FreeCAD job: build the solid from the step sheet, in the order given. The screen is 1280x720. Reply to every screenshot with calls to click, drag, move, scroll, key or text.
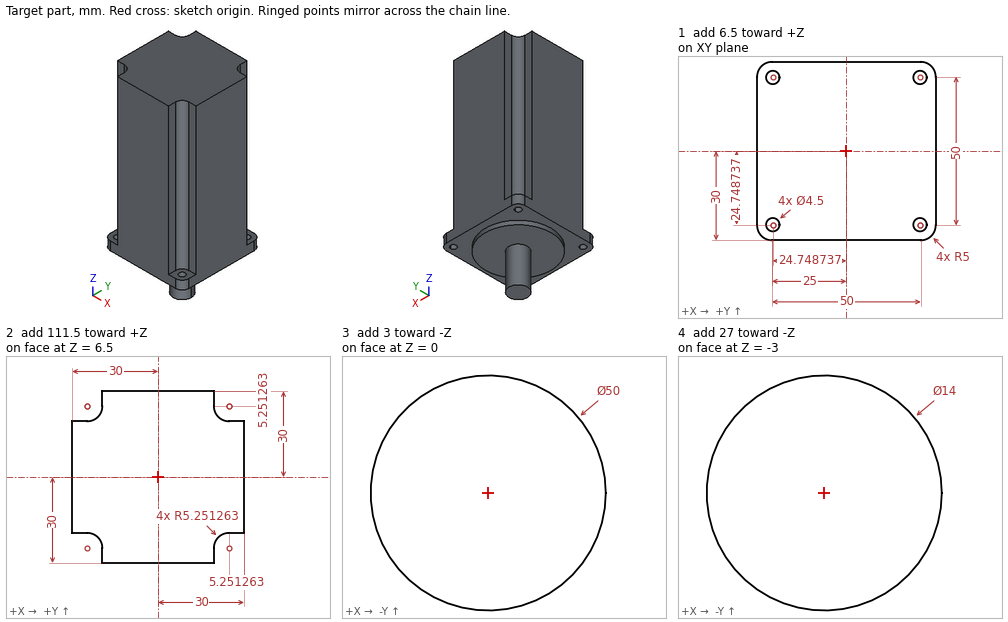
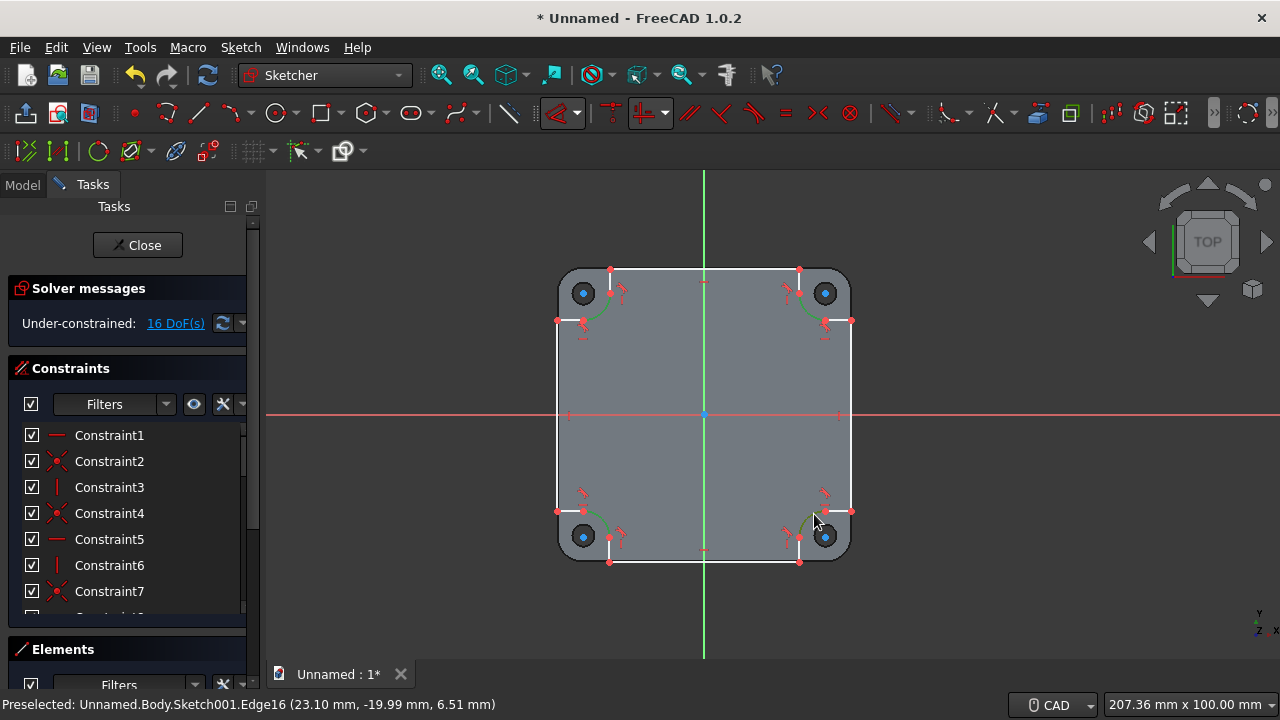
key(e)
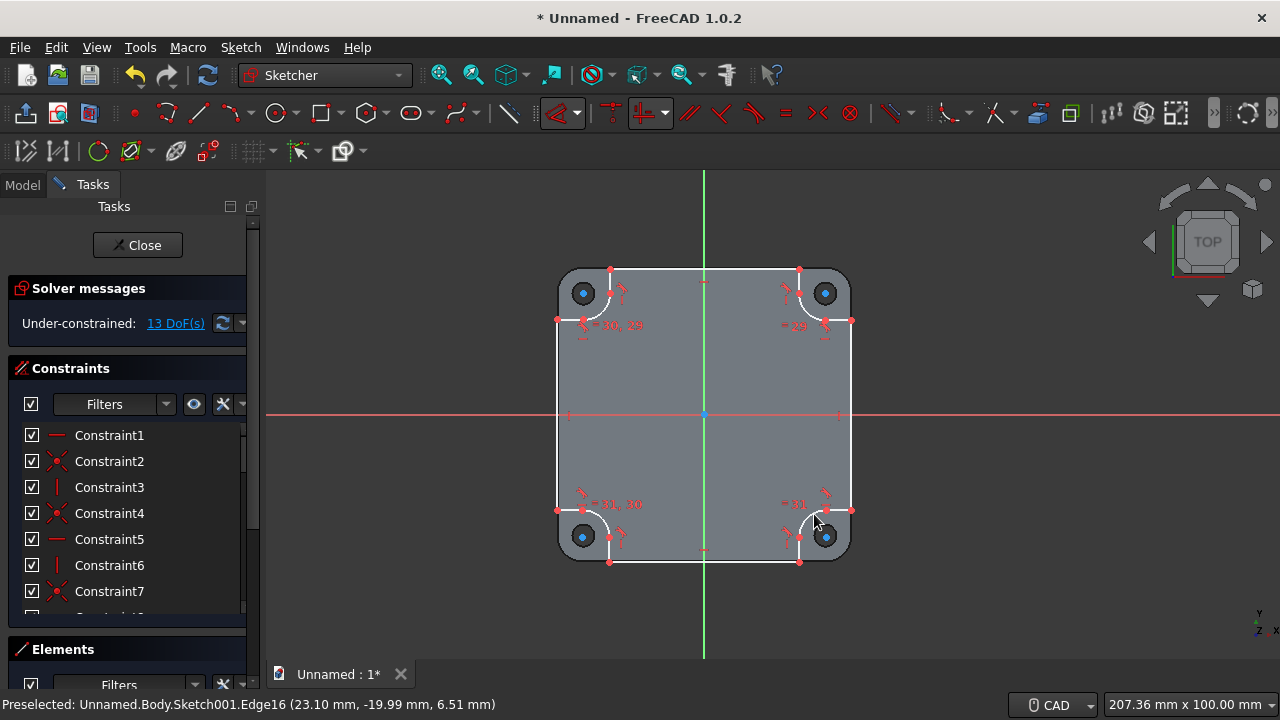
click(826, 294)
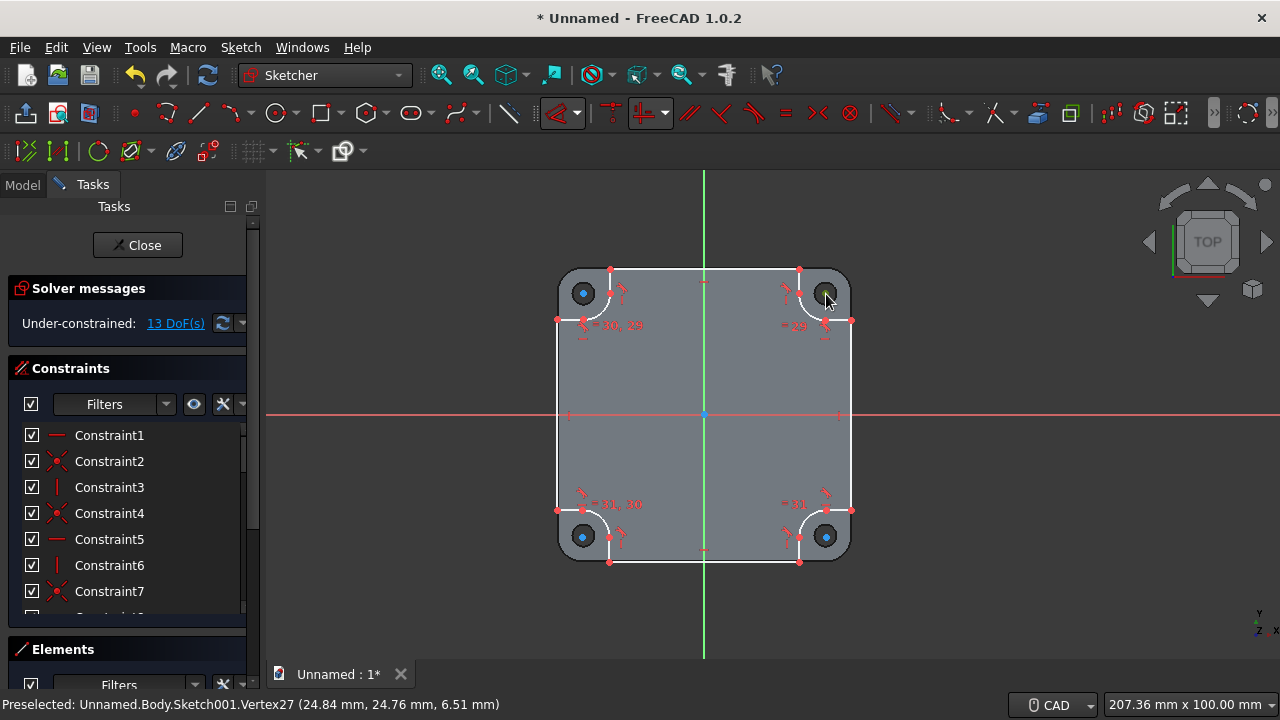
click(583, 293)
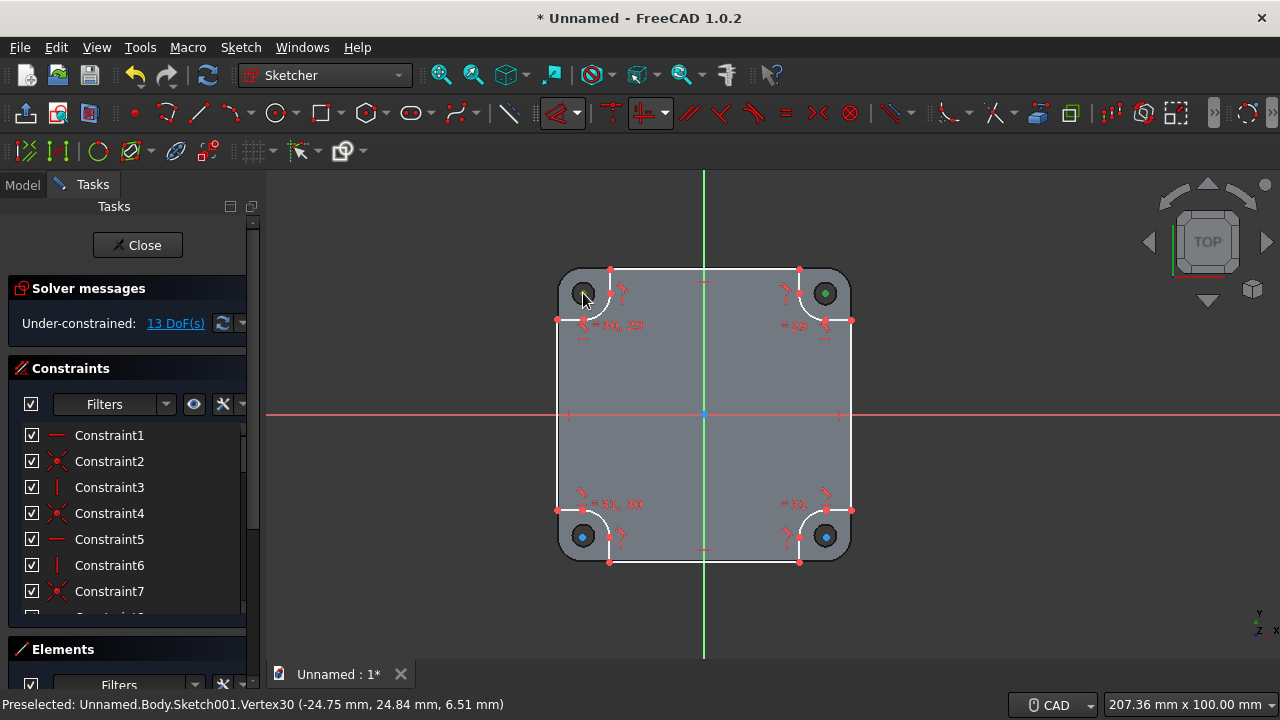
click(704, 600)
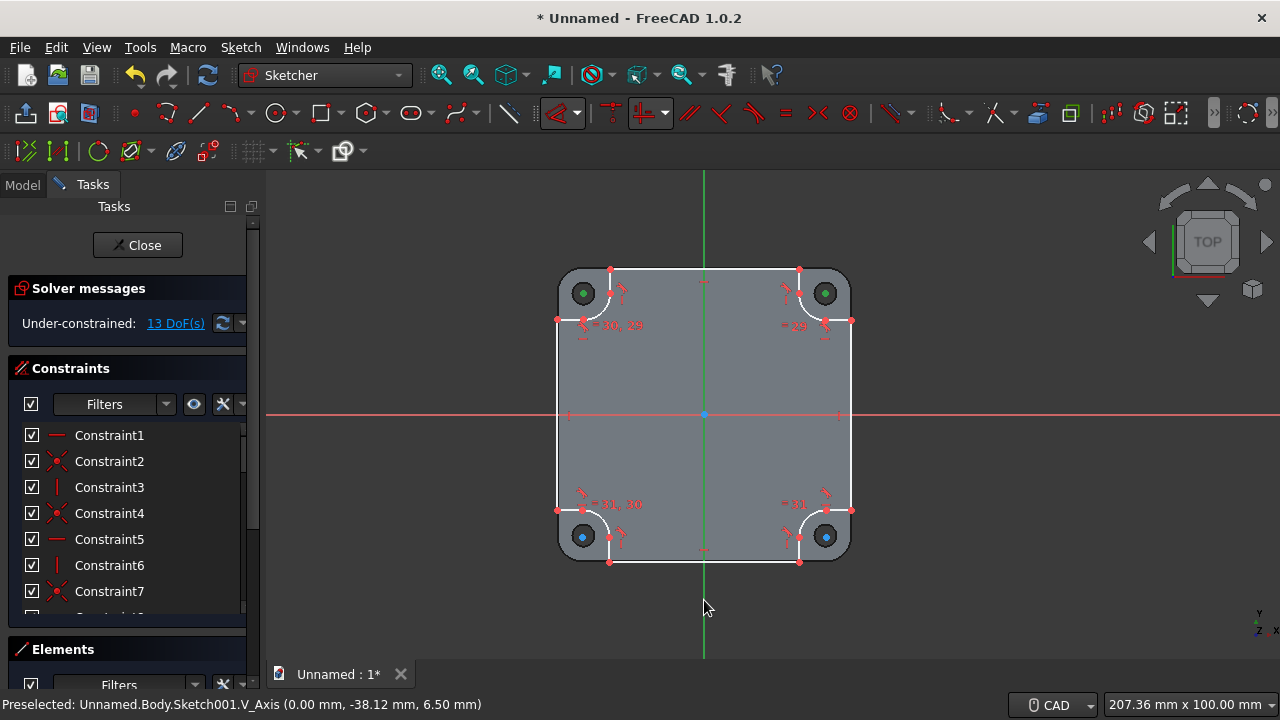
click(818, 114)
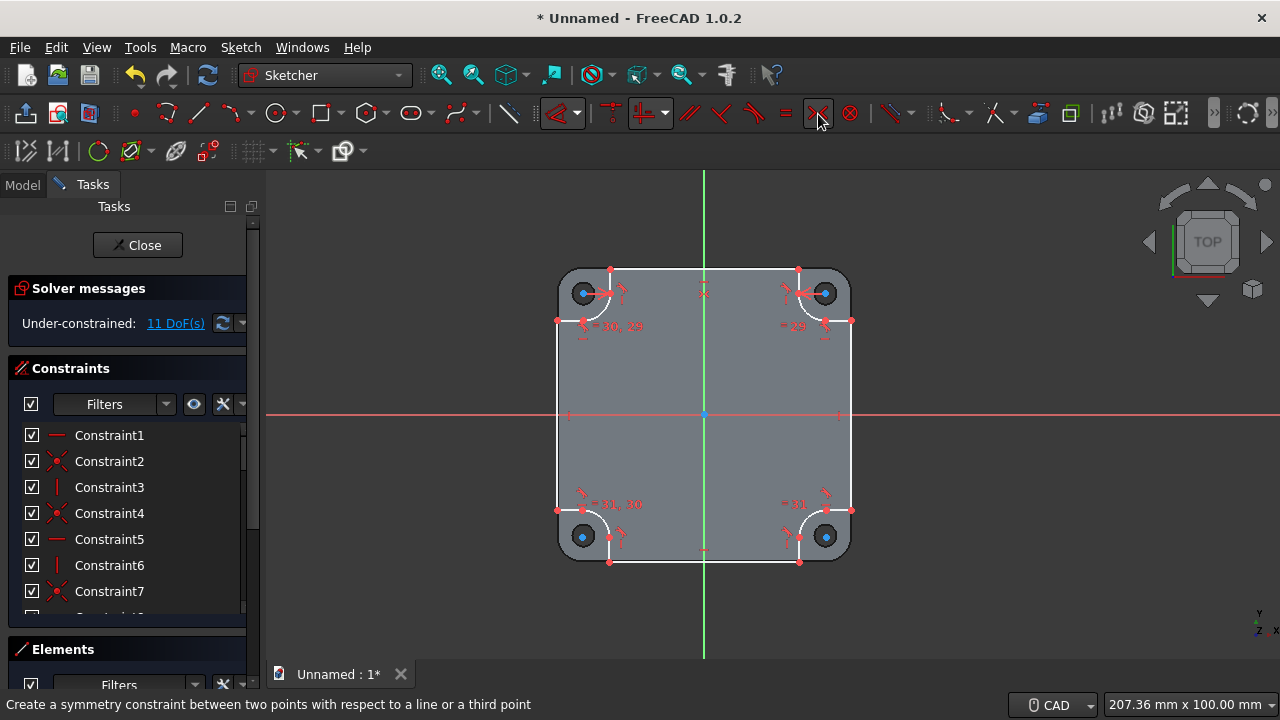
click(583, 294)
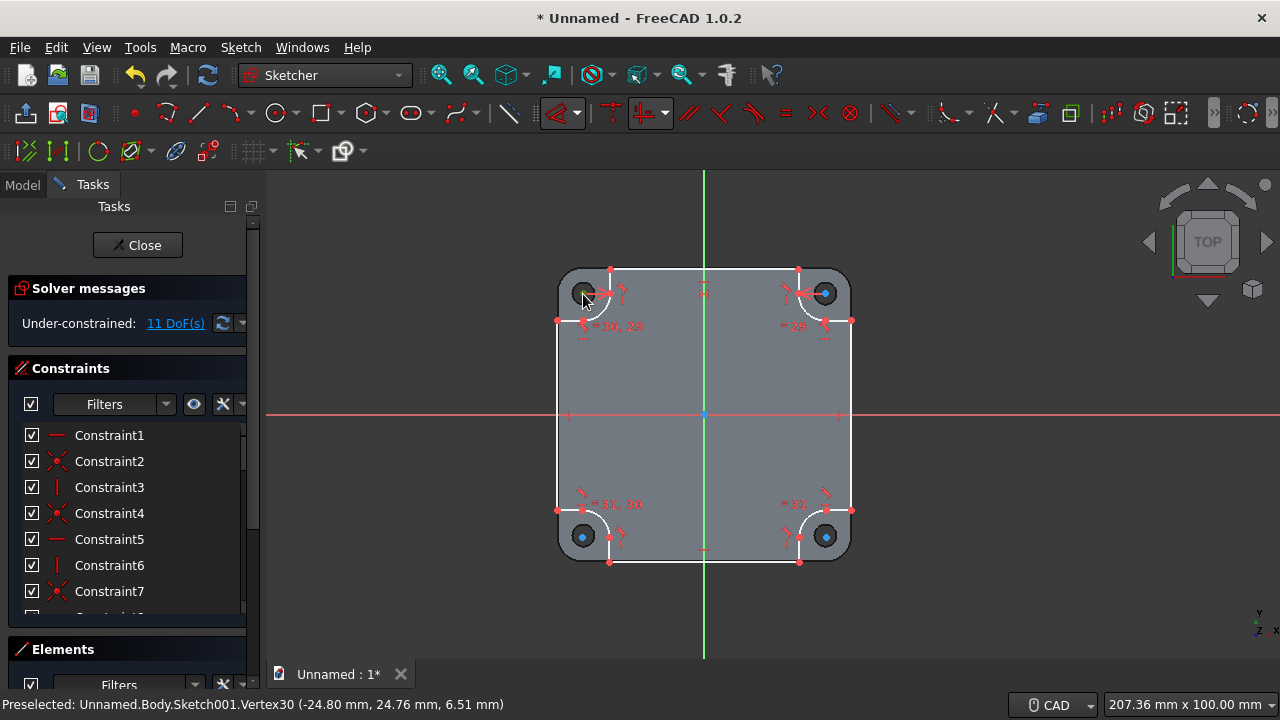
click(582, 537)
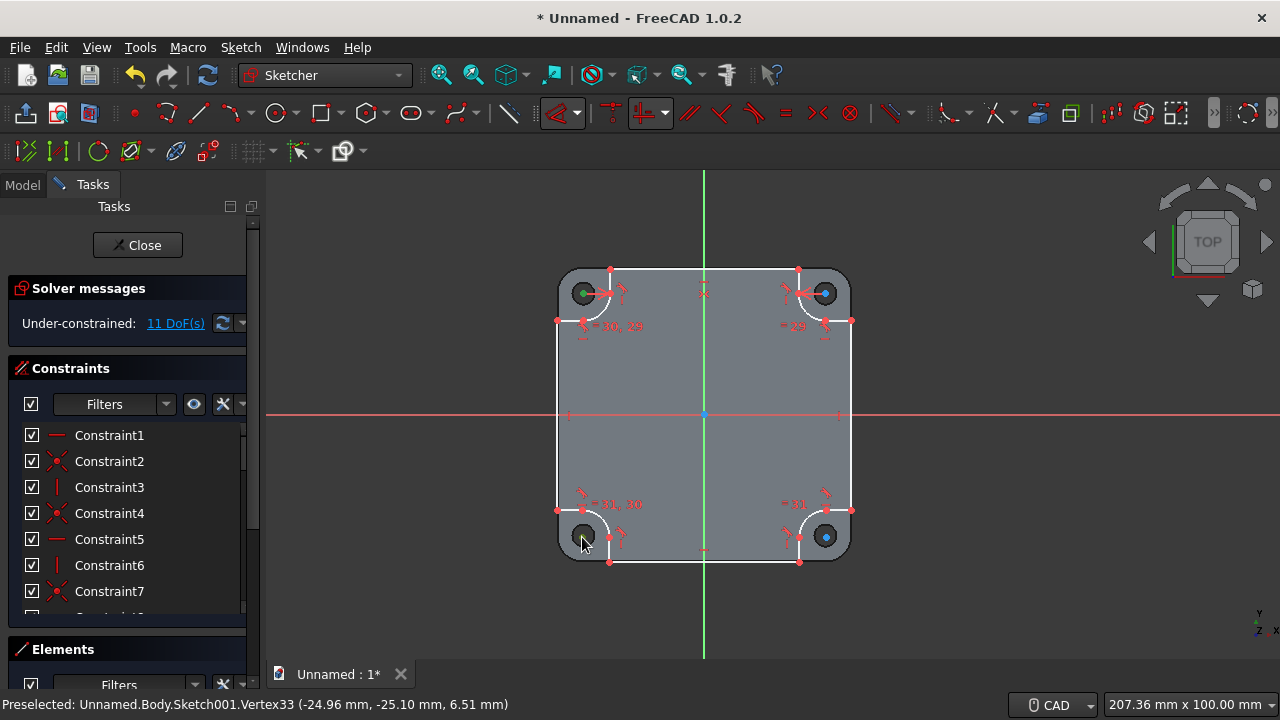
click(353, 415)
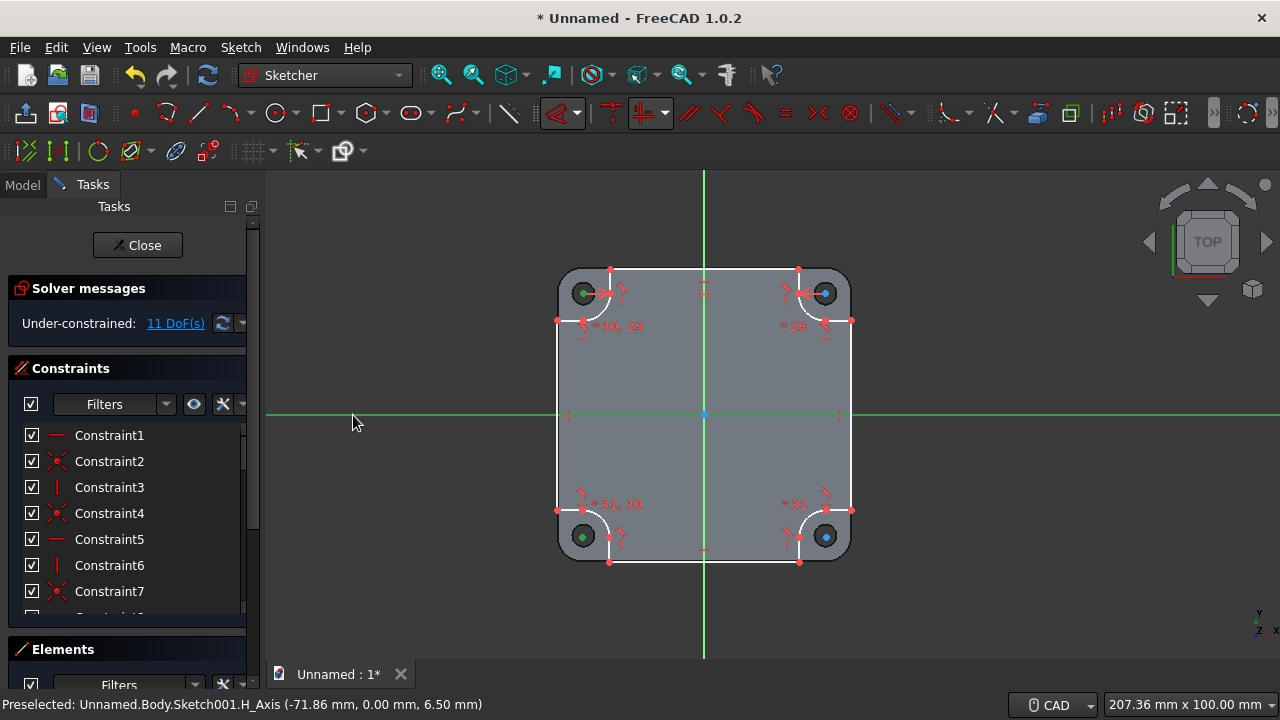
key(s)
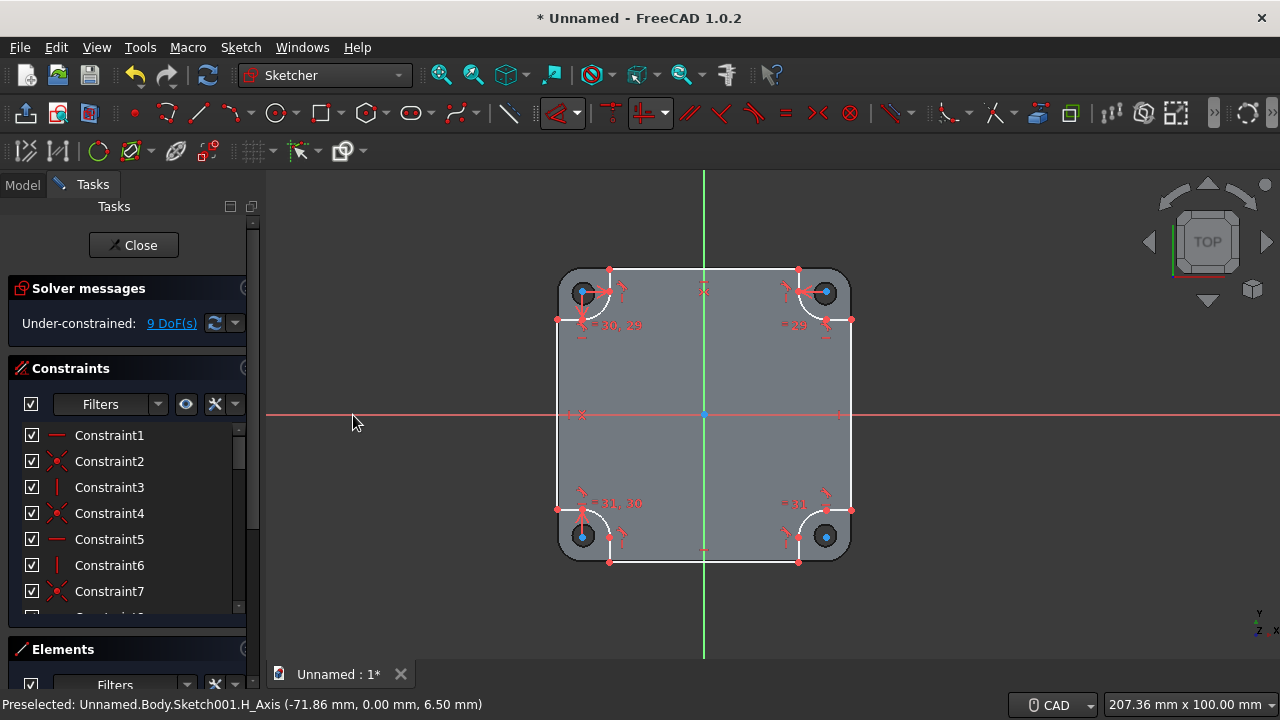
click(826, 292)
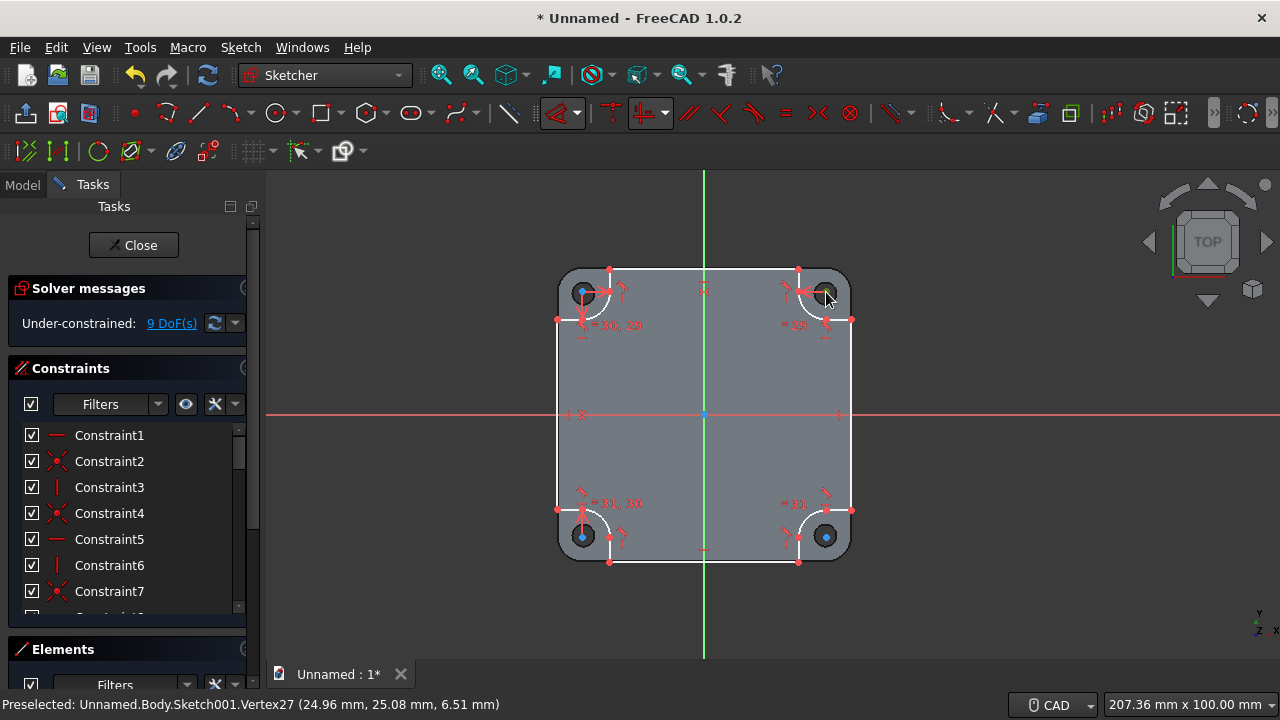
click(826, 538)